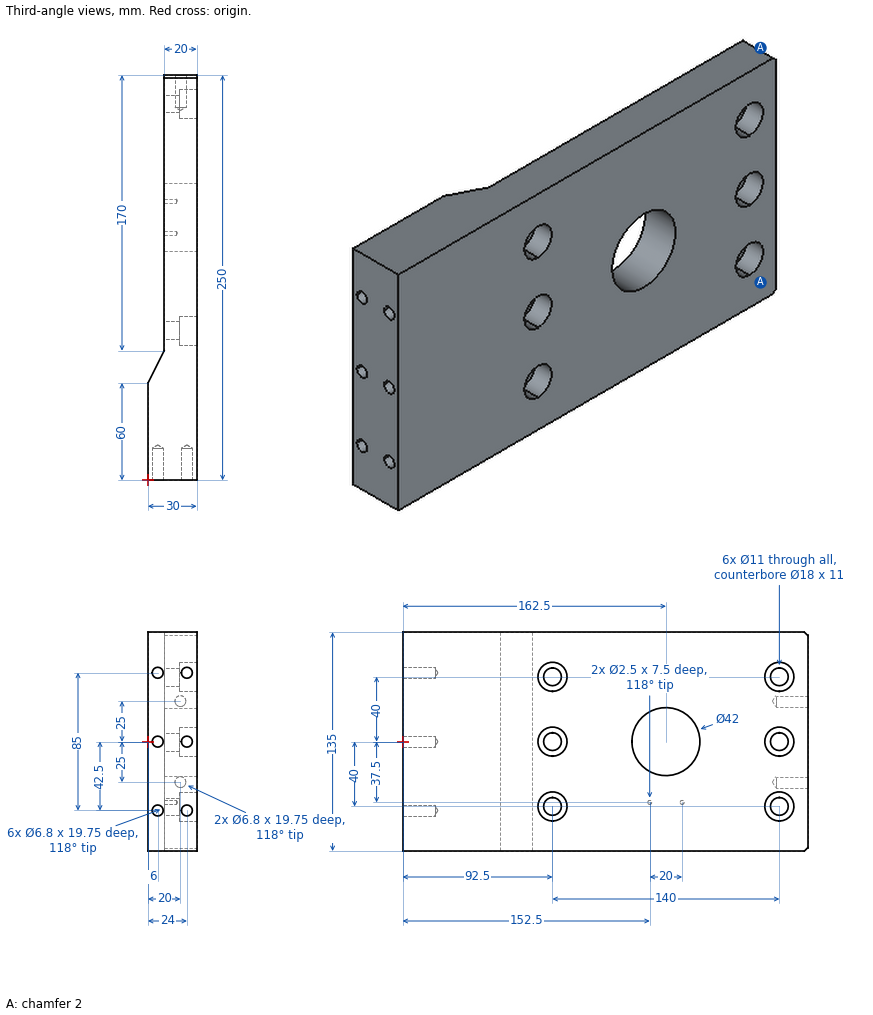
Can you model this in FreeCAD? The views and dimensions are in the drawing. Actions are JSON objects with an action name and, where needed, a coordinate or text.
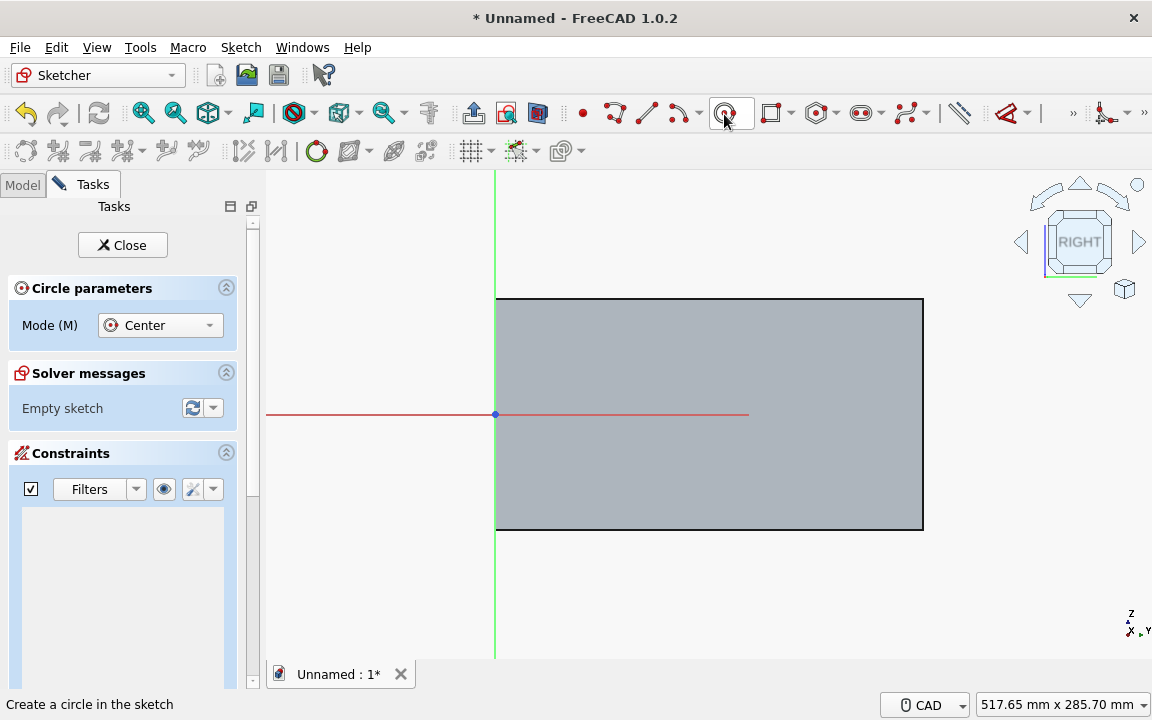
{"action": "scroll", "coordinate": [893, 346], "scroll_direction": "up", "scroll_amount": 5}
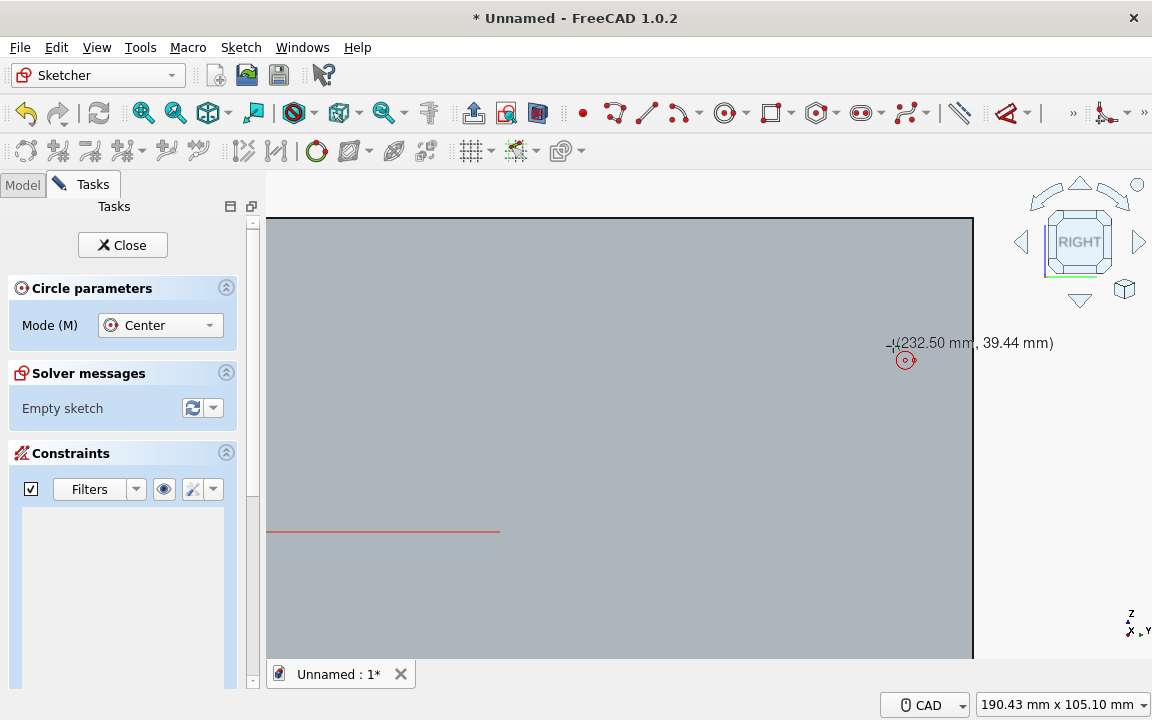
{"action": "left_click", "coordinate": [892, 345]}
{"action": "mouse_move", "coordinate": [910, 327]}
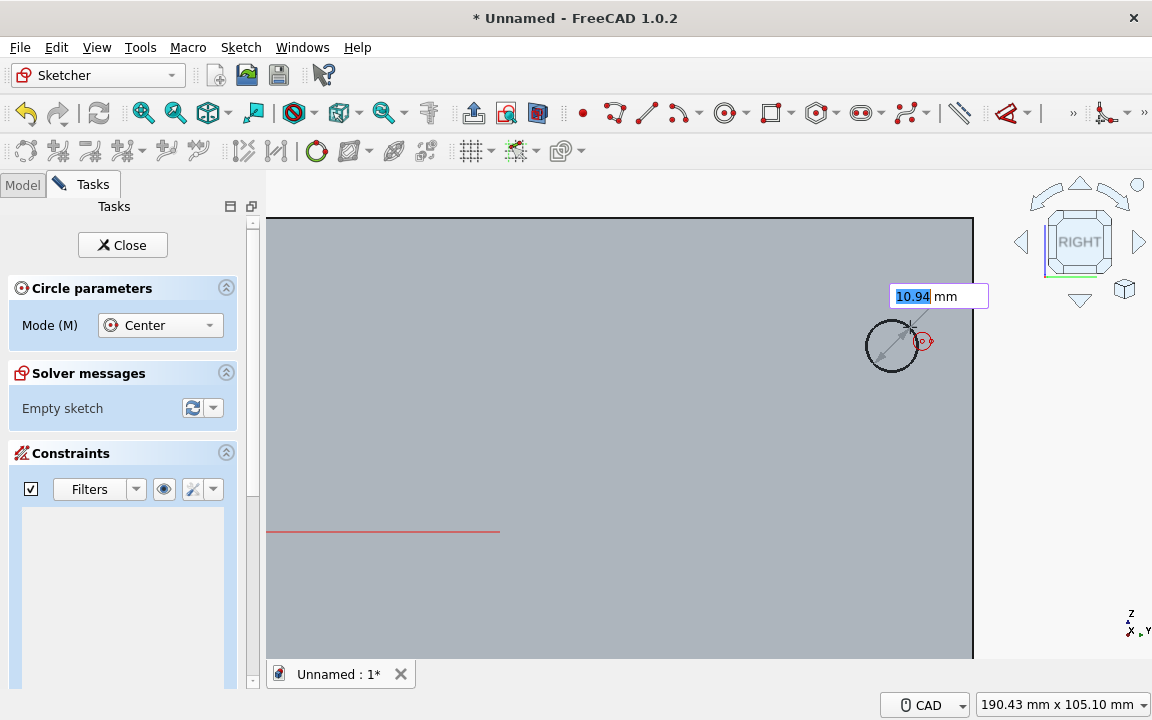
{"action": "type", "text": "11"}
{"action": "key", "text": "Return"}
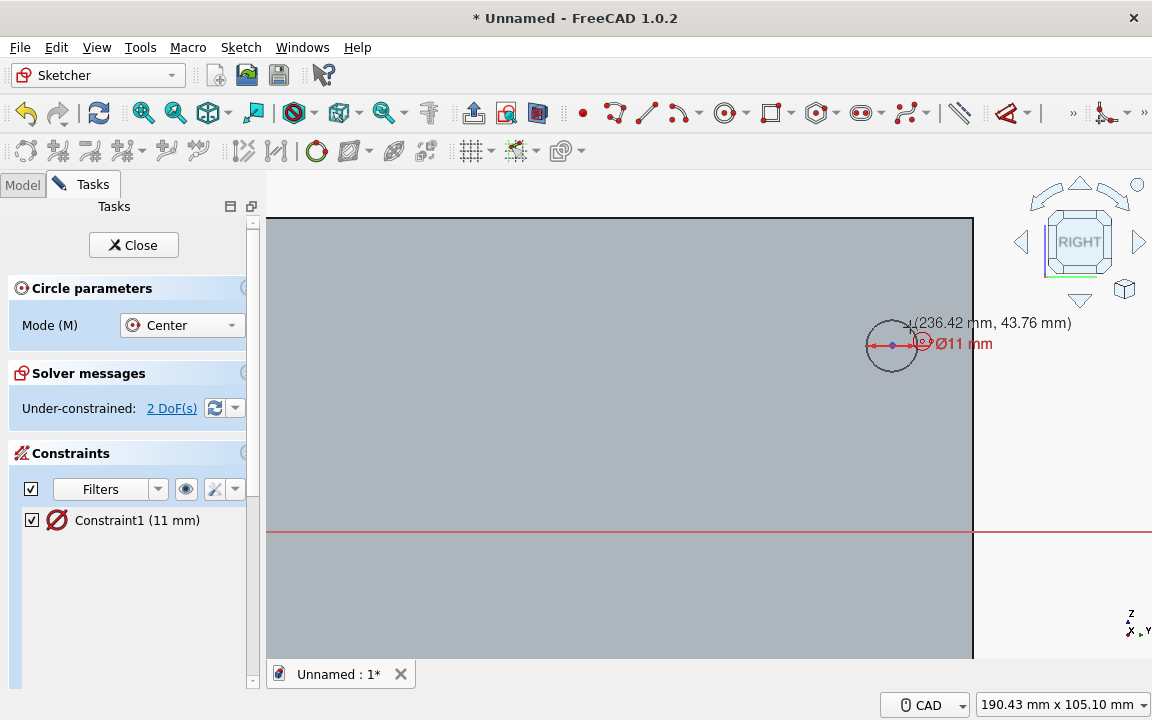
{"action": "scroll", "coordinate": [866, 319], "scroll_direction": "down", "scroll_amount": 4}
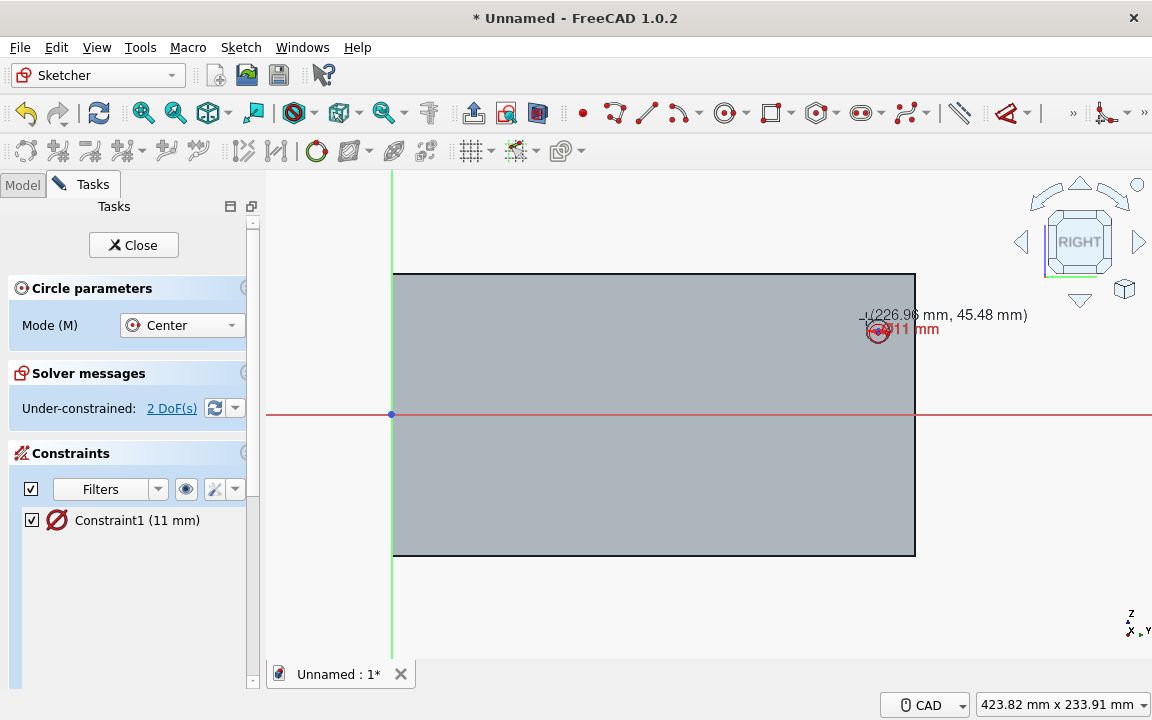
{"action": "scroll", "coordinate": [878, 498], "scroll_direction": "up", "scroll_amount": 4}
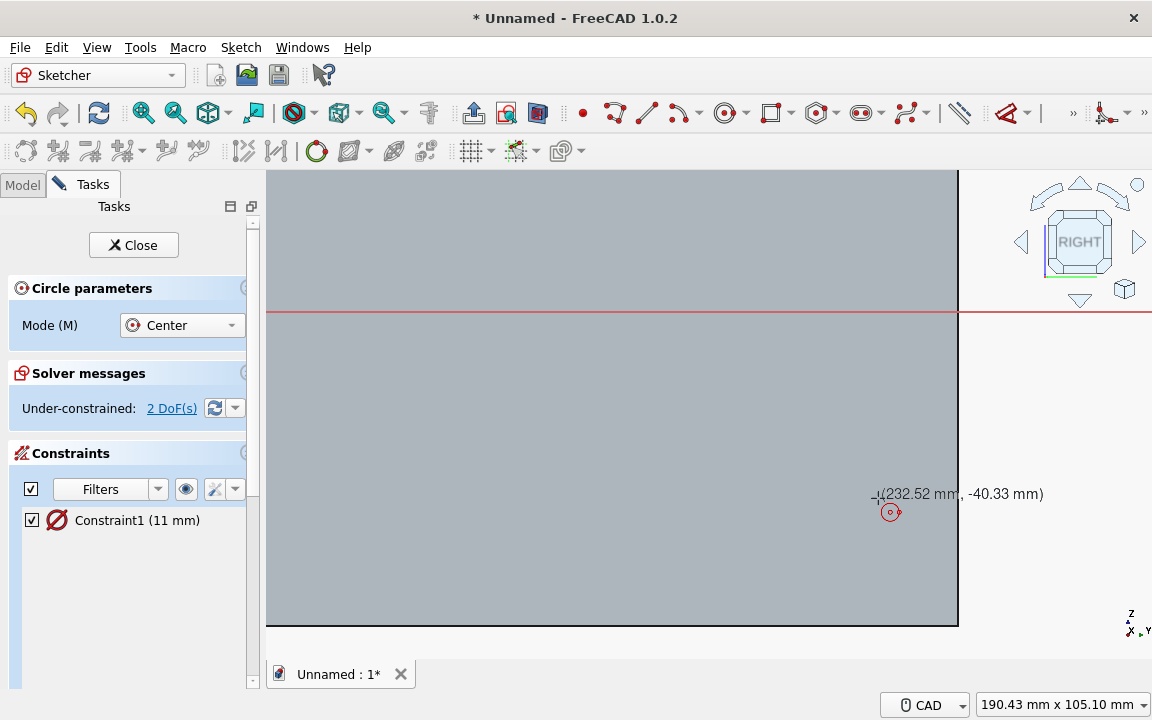
{"action": "left_click", "coordinate": [877, 498]}
{"action": "mouse_move", "coordinate": [895, 480]}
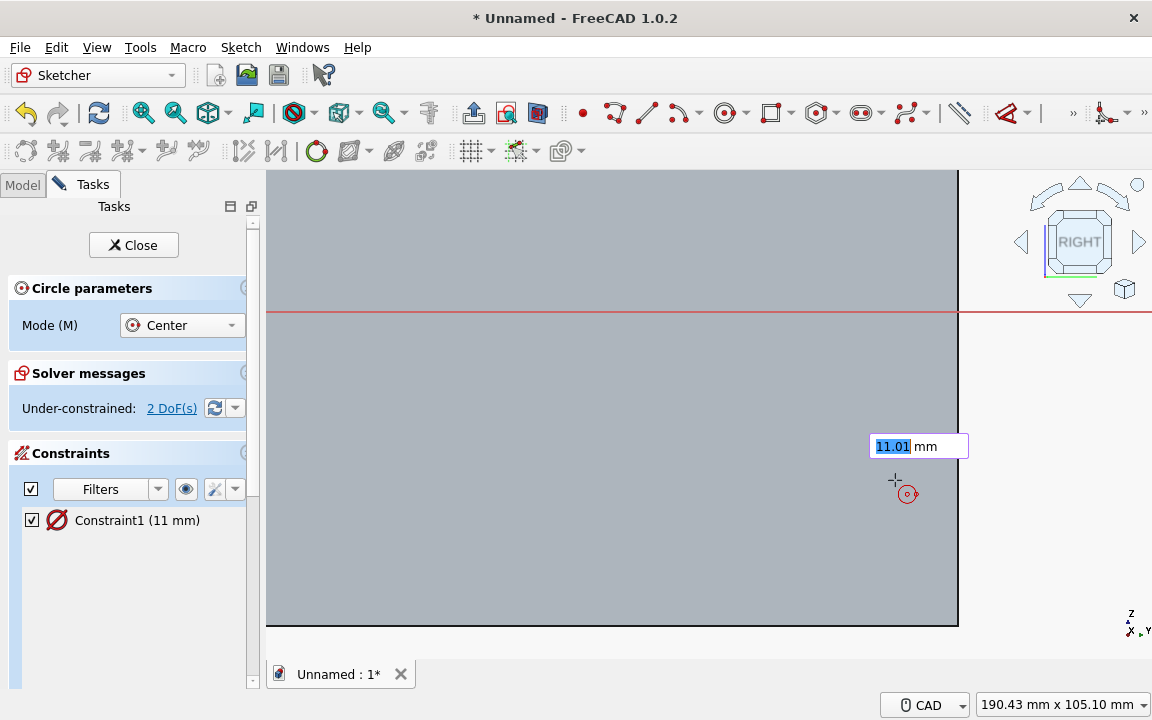
{"action": "type", "text": "11"}
{"action": "key", "text": "Return"}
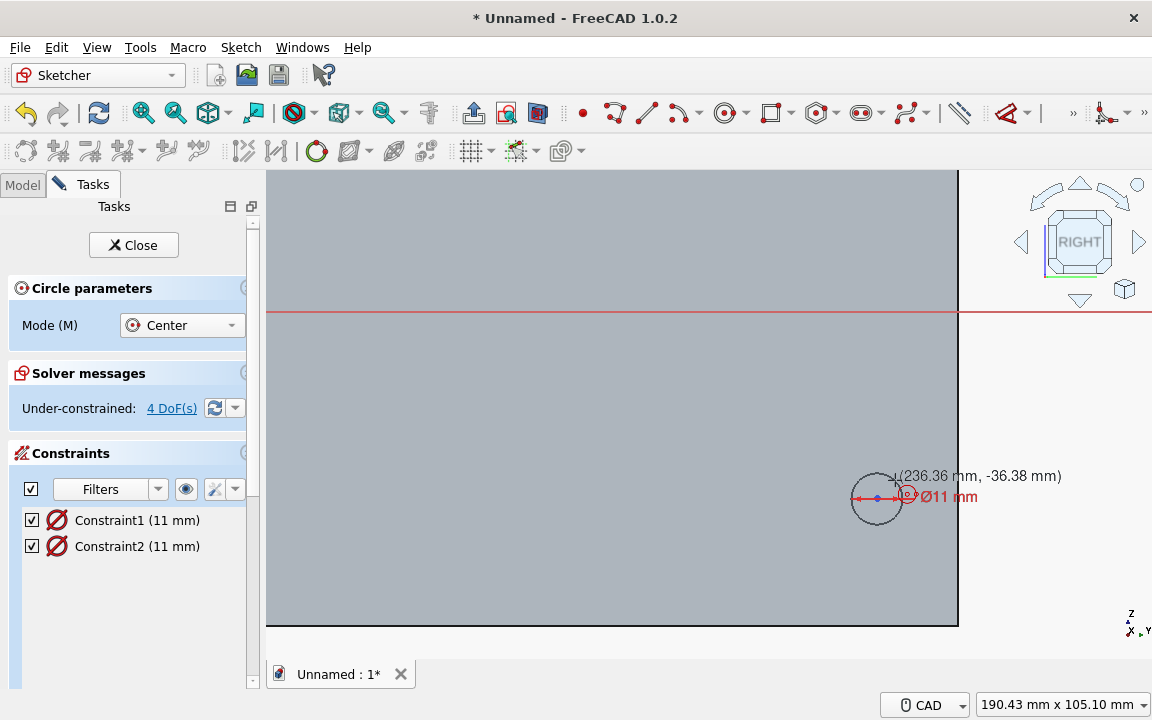
{"action": "scroll", "coordinate": [878, 498], "scroll_direction": "down", "scroll_amount": 4}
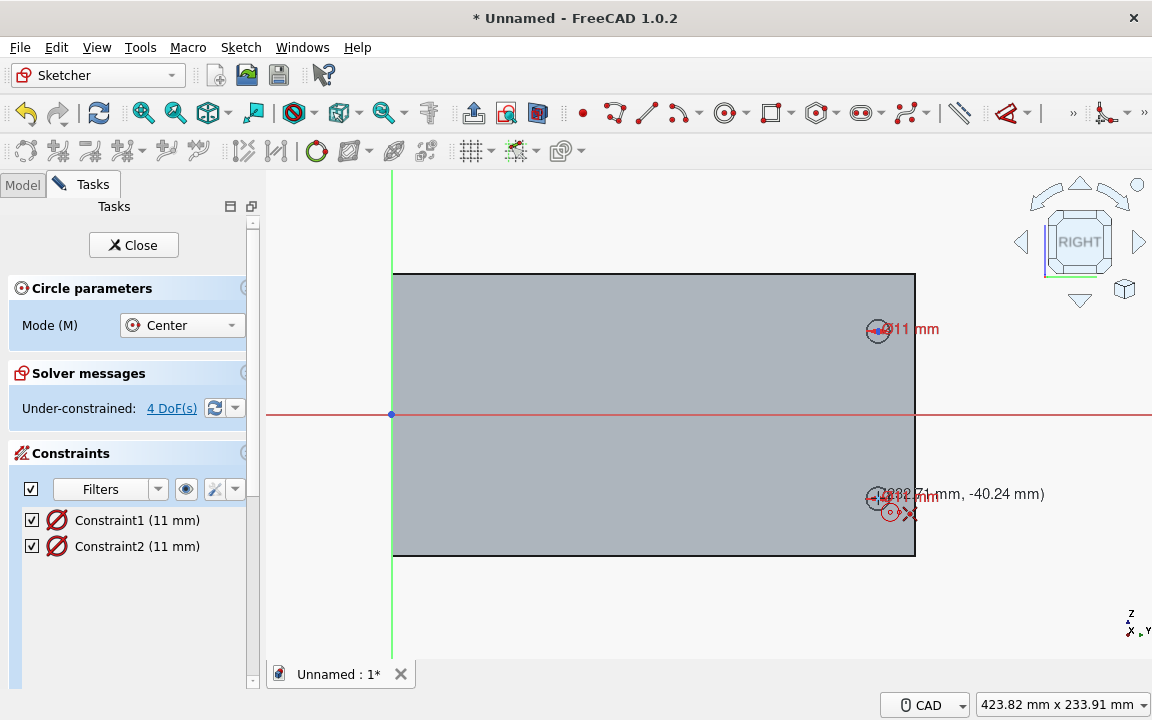
{"action": "scroll", "coordinate": [585, 498], "scroll_direction": "up", "scroll_amount": 4}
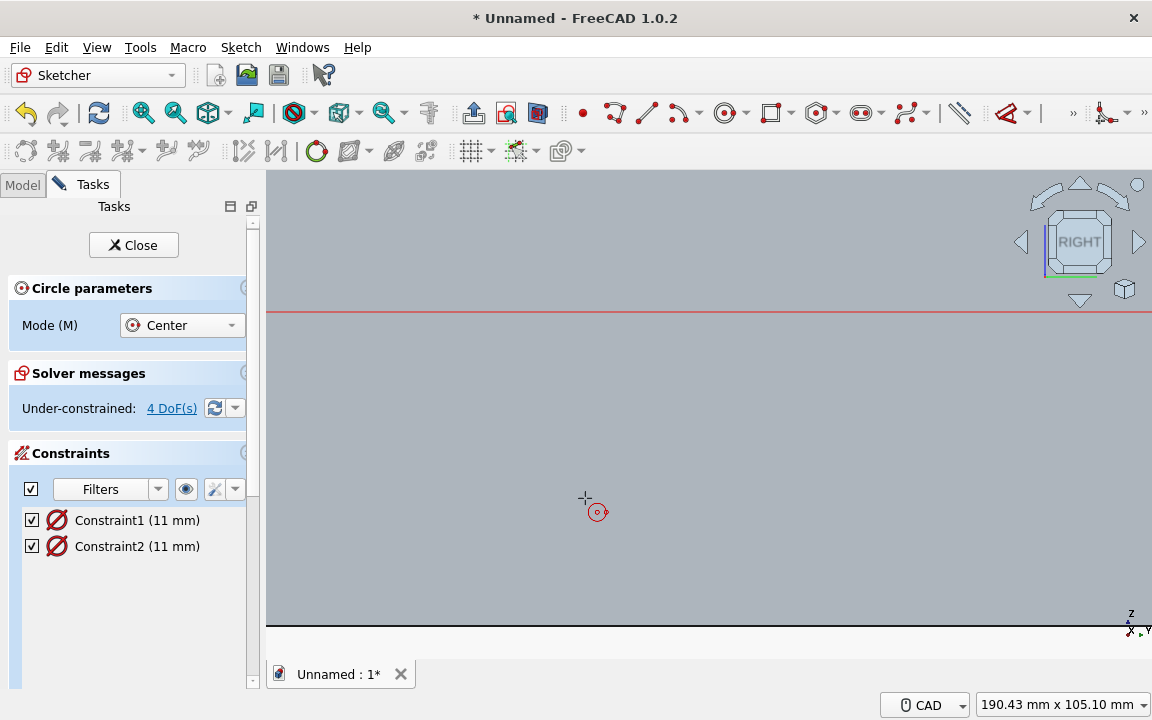
{"action": "left_click", "coordinate": [585, 498]}
{"action": "mouse_move", "coordinate": [603, 480]}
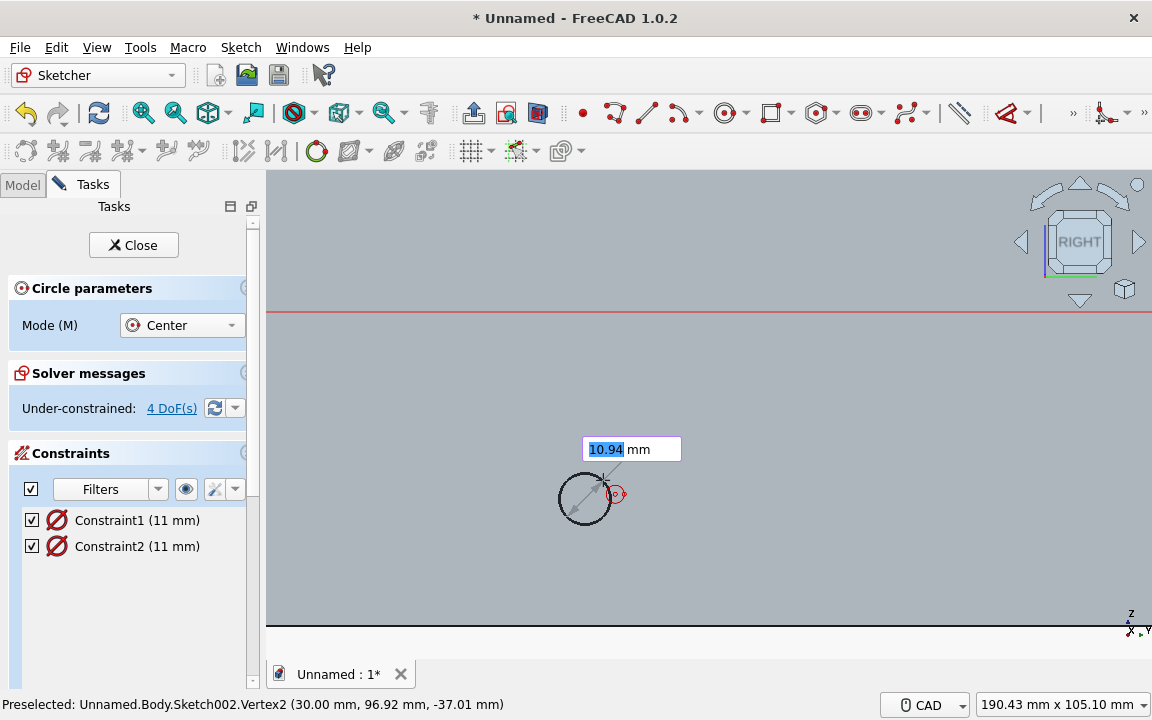
{"action": "type", "text": "11"}
{"action": "key", "text": "Return"}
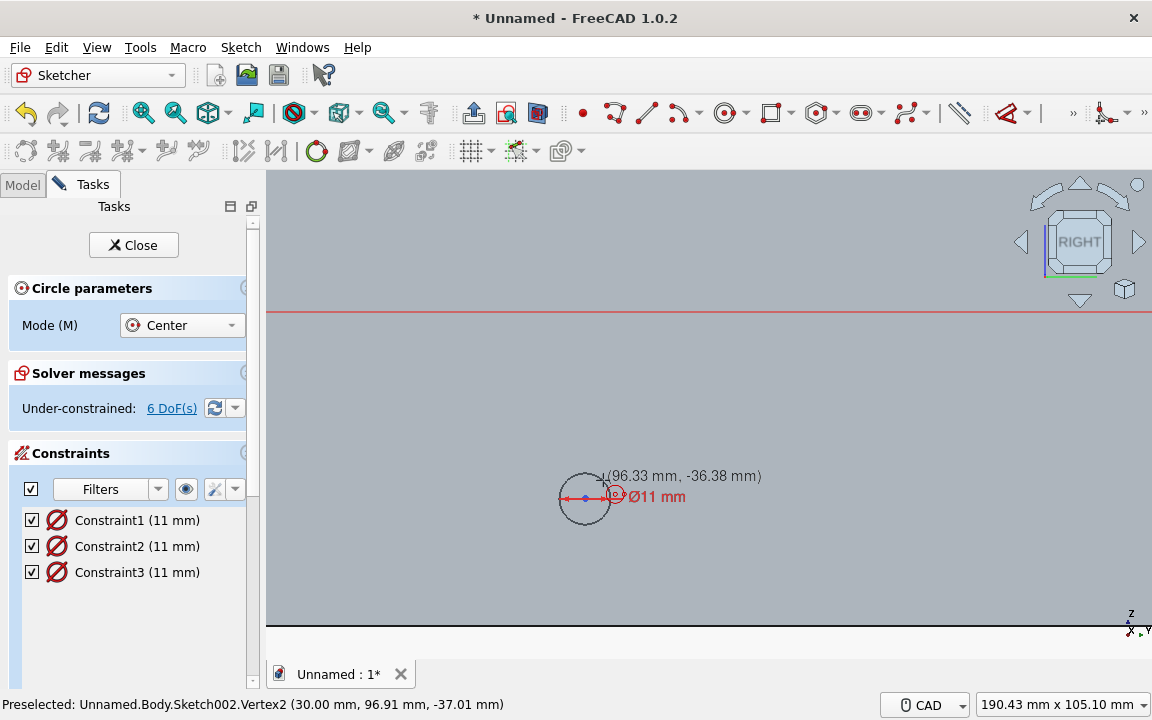
{"action": "scroll", "coordinate": [585, 498], "scroll_direction": "down", "scroll_amount": 4}